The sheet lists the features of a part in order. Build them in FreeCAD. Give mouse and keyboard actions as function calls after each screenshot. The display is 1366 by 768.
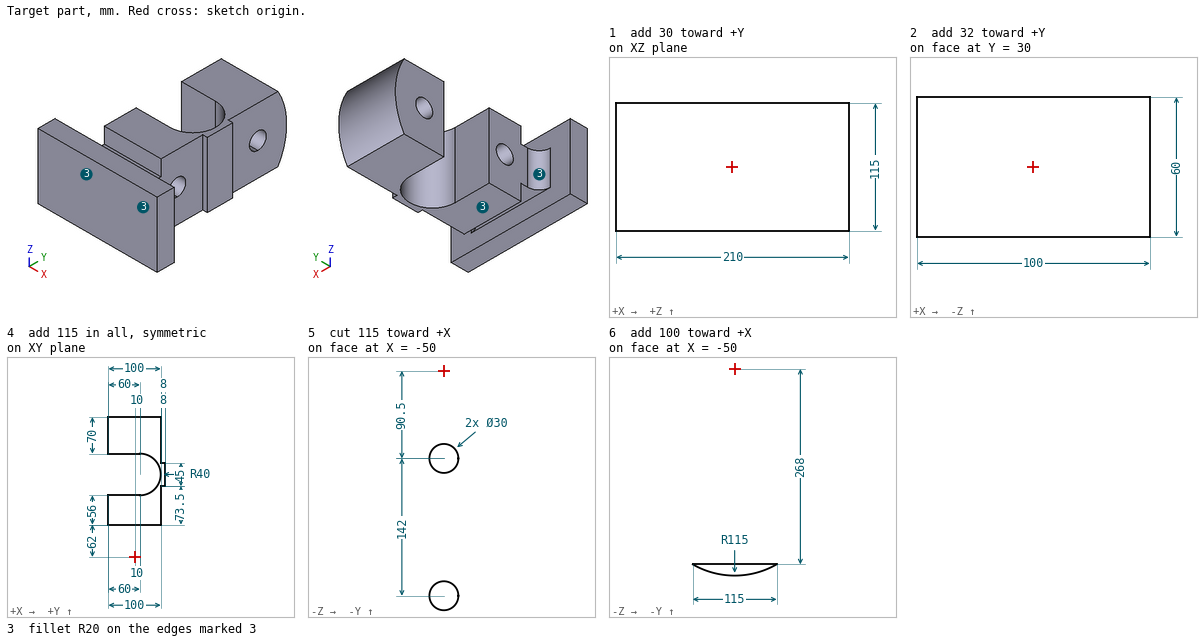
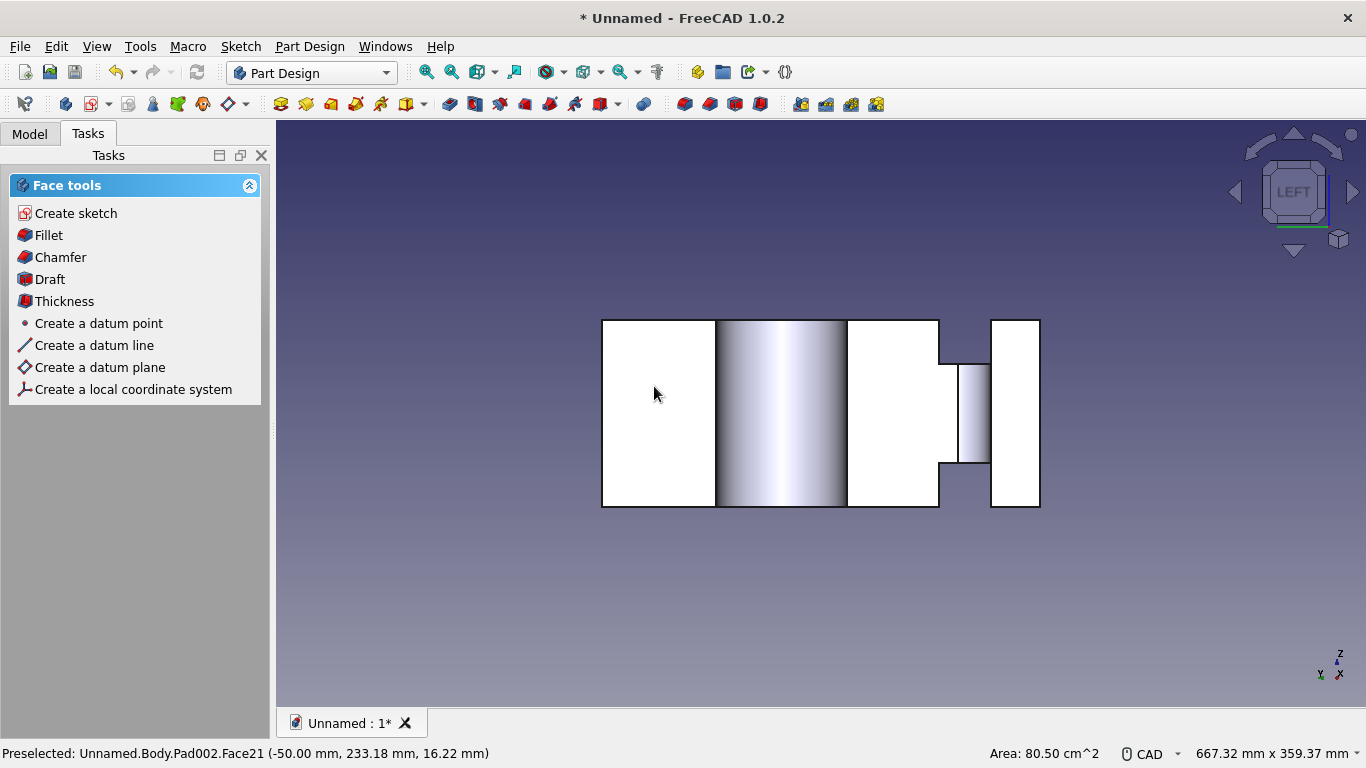
click(90, 104)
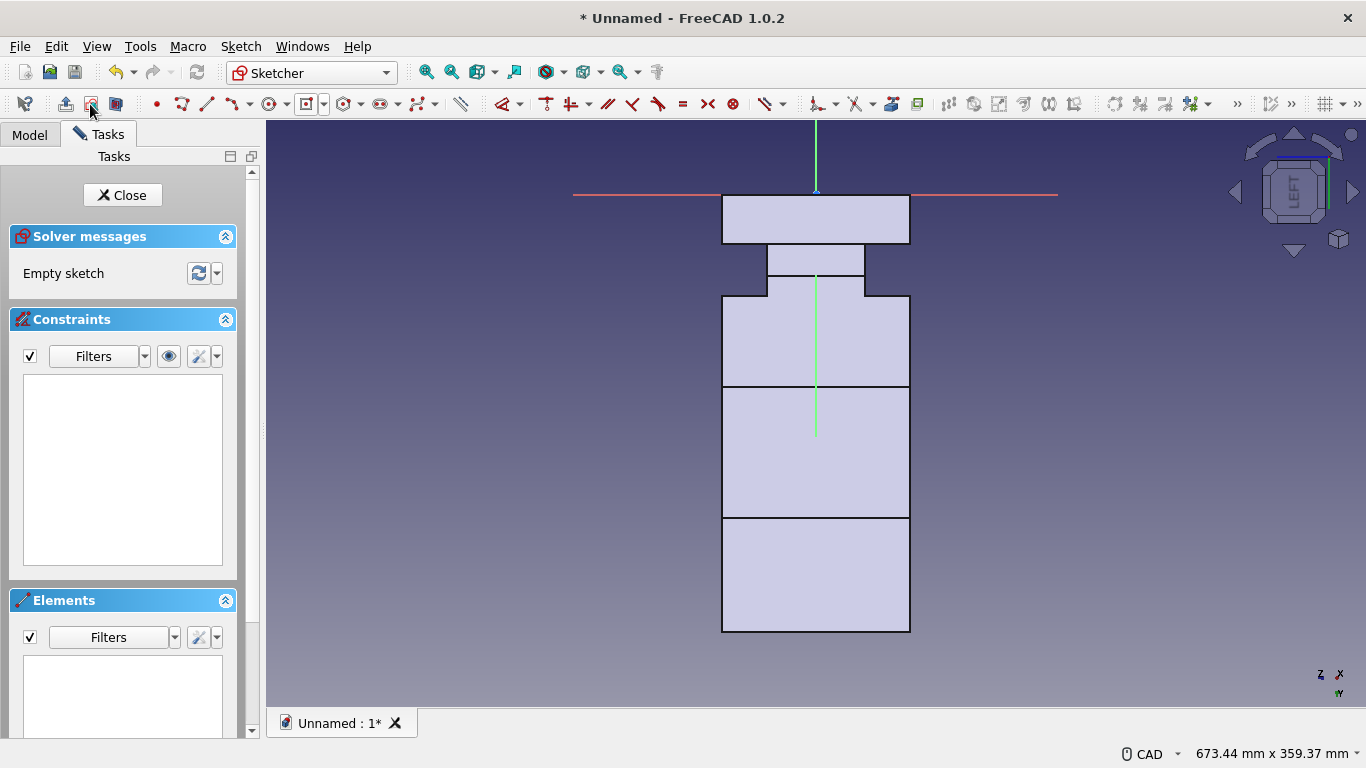
click(268, 104)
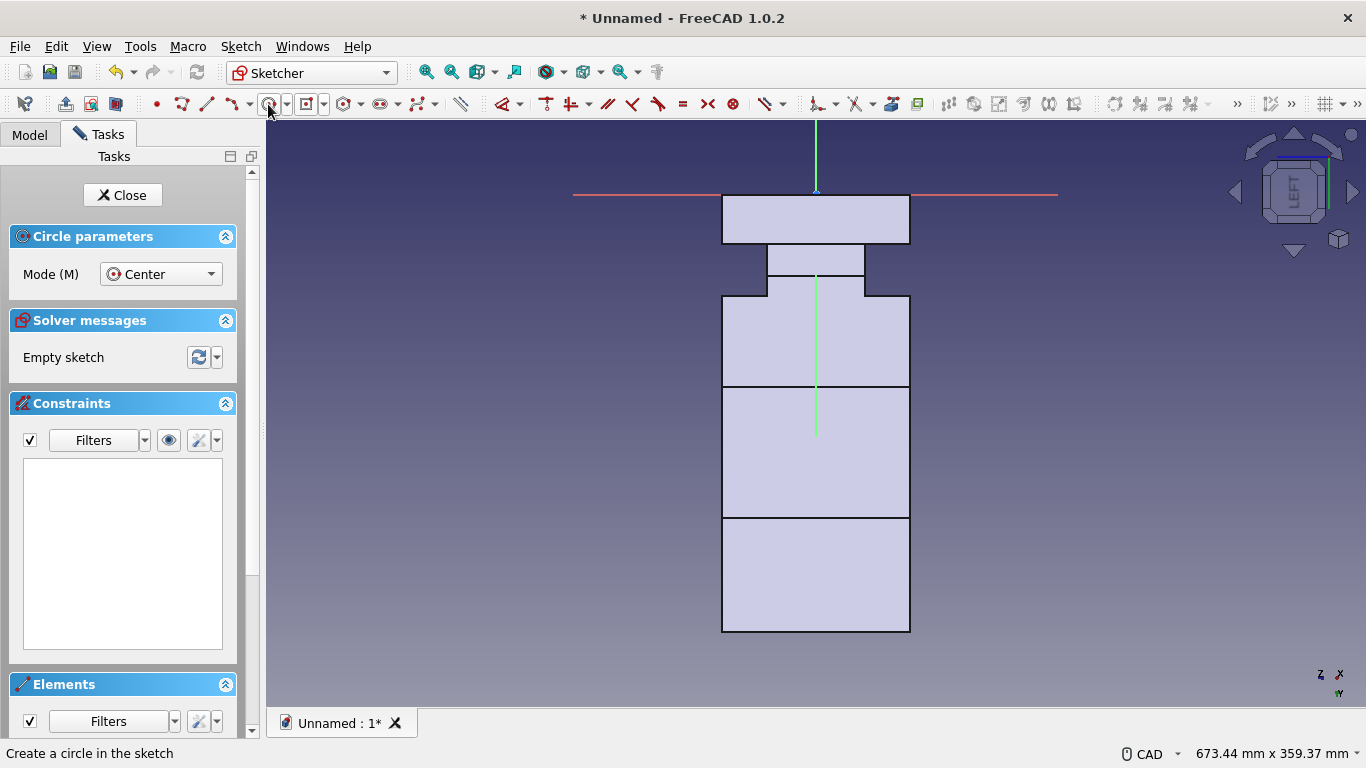
click(816, 342)
move(833, 325)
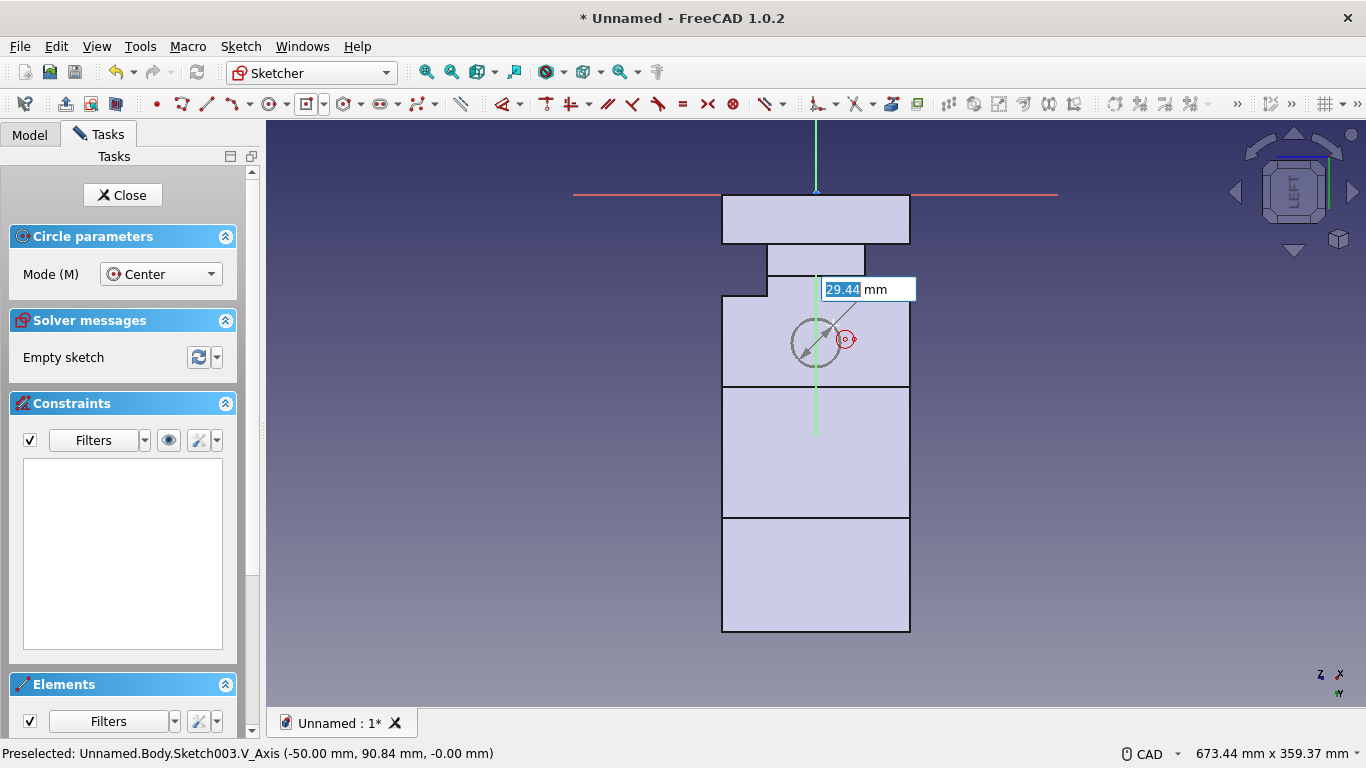
text(30)
key(Return)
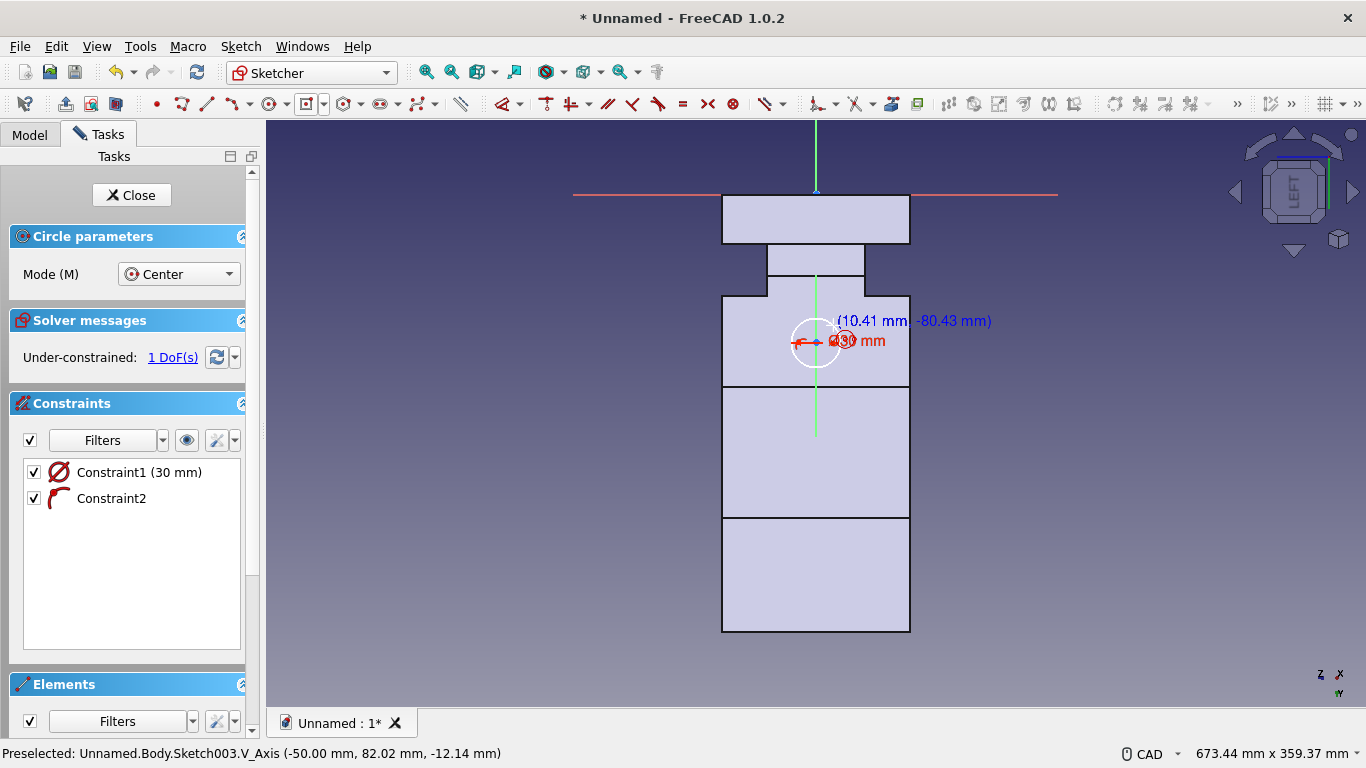
click(816, 574)
move(833, 557)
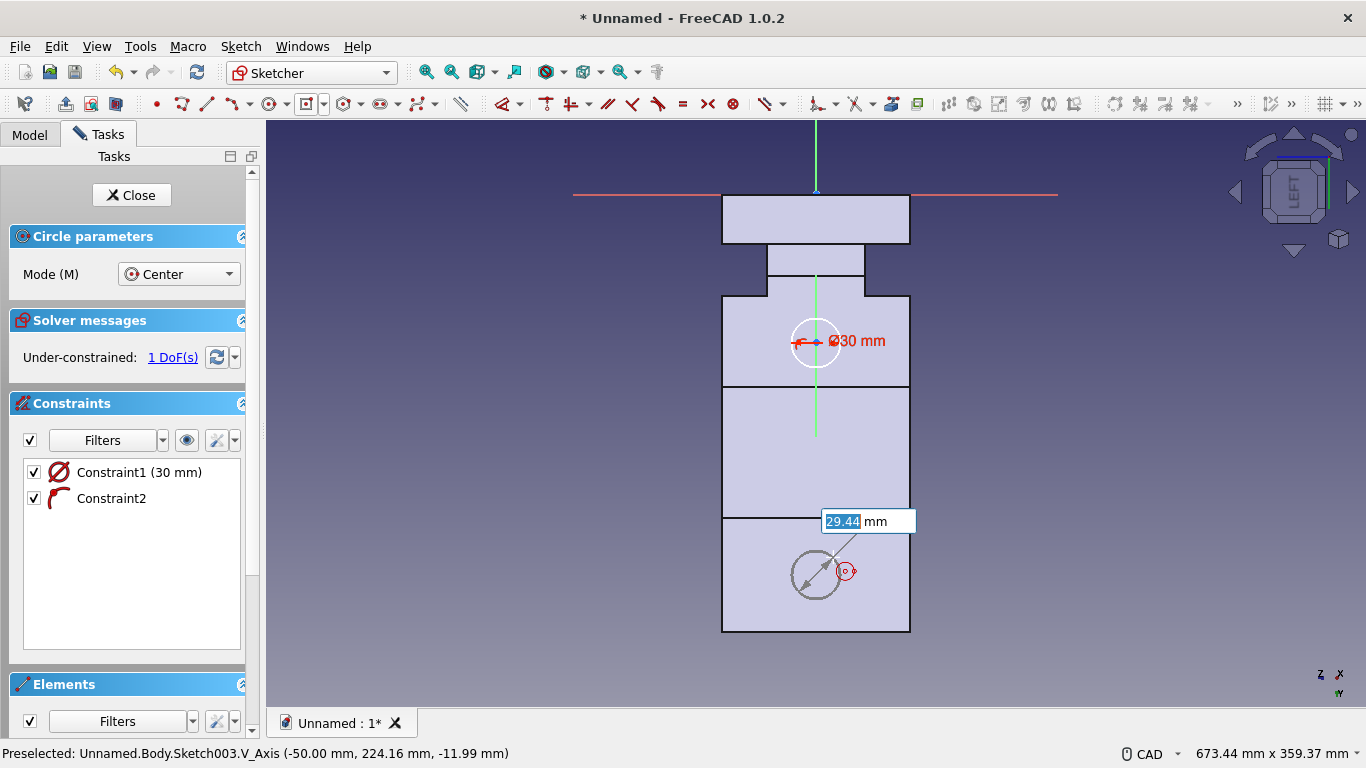
text(30)
key(Return)
key(Escape)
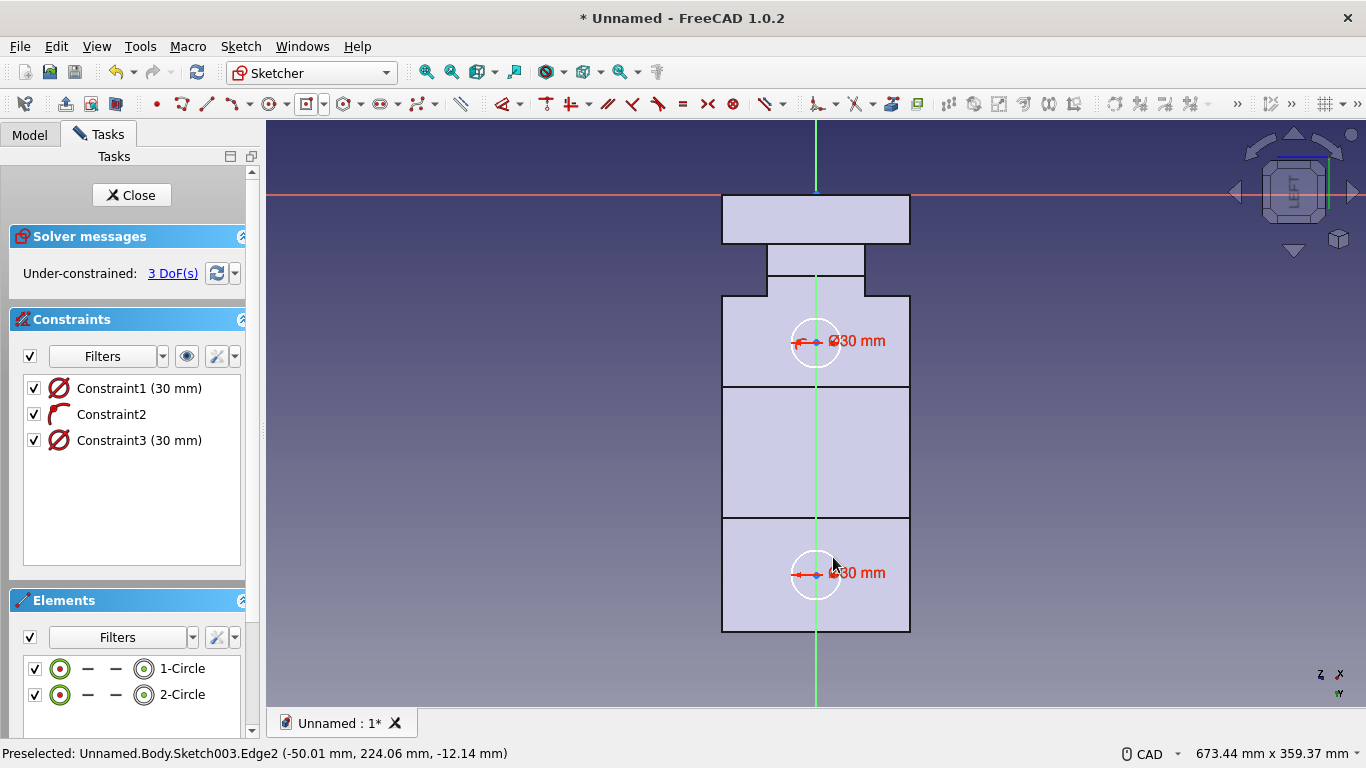
click(816, 575)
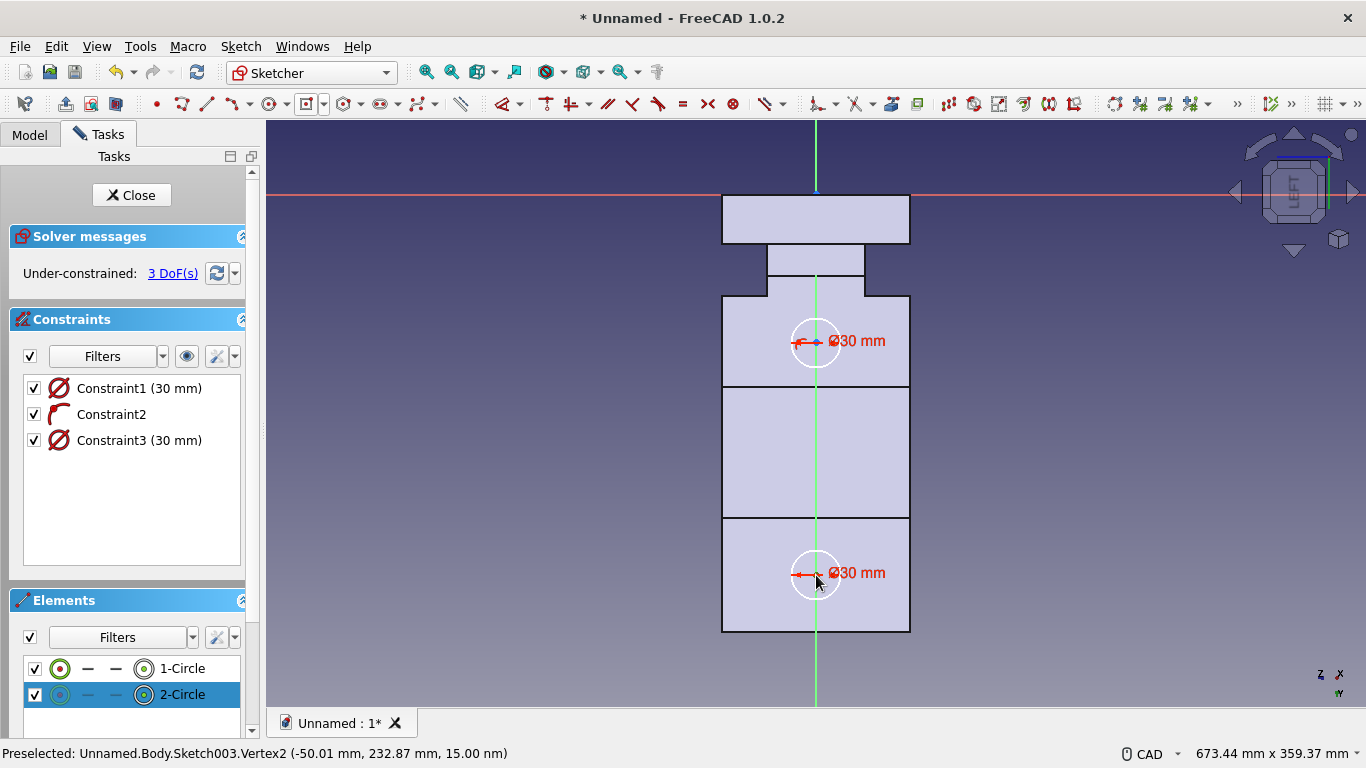
click(816, 641)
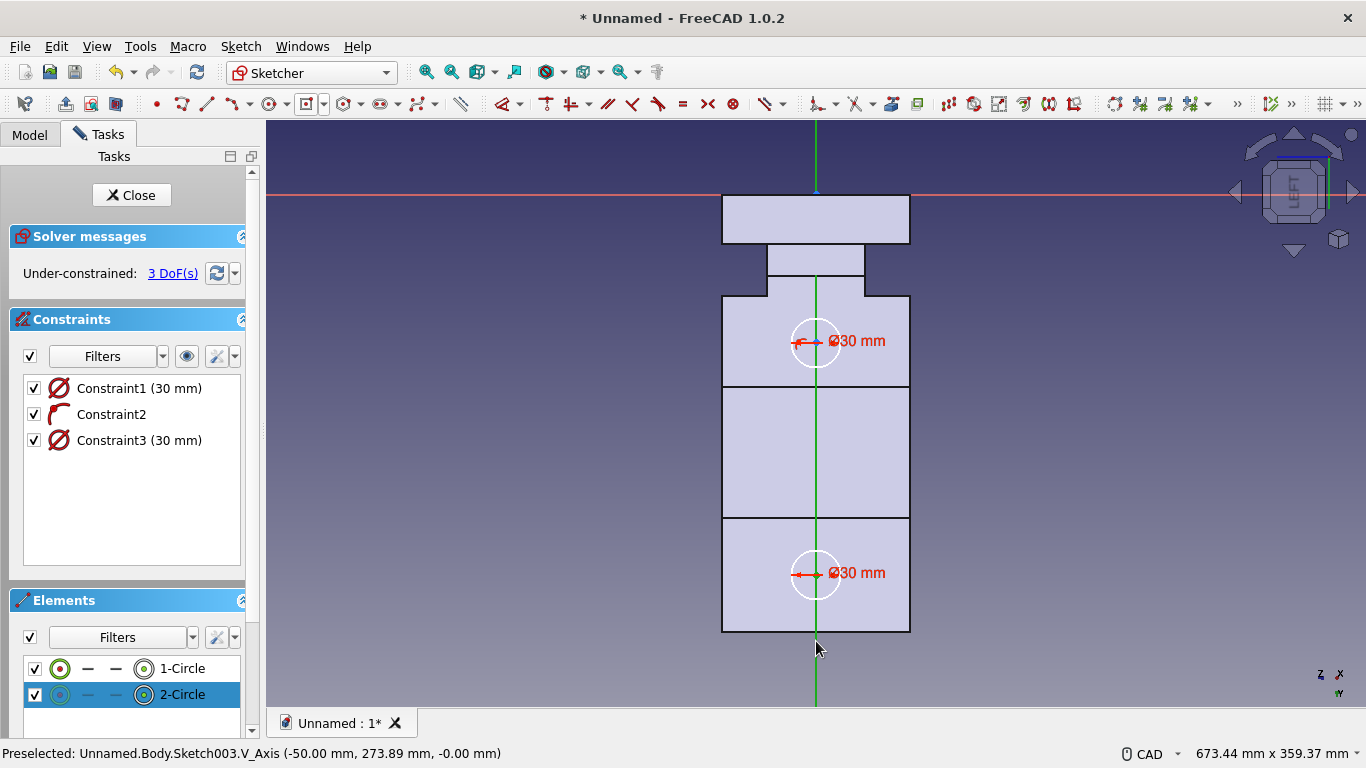
key(c)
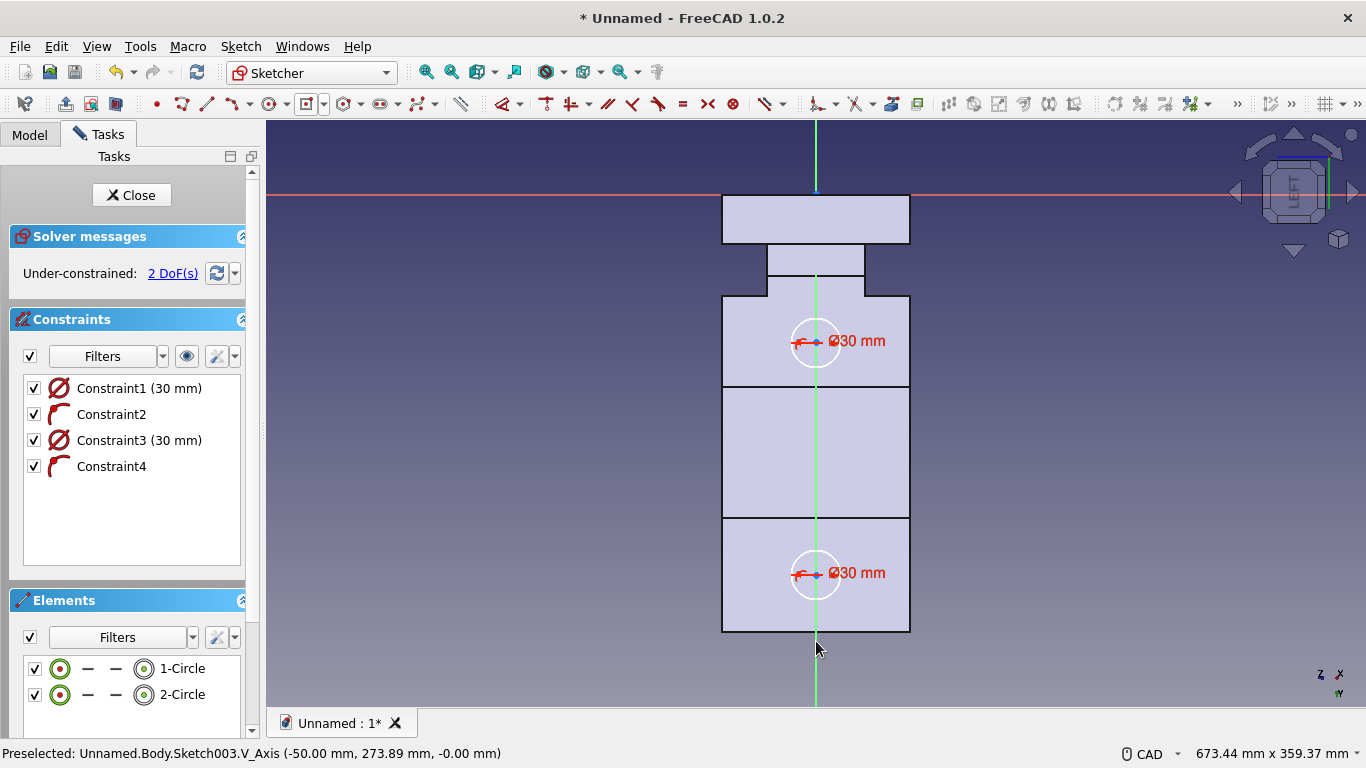
key(d)